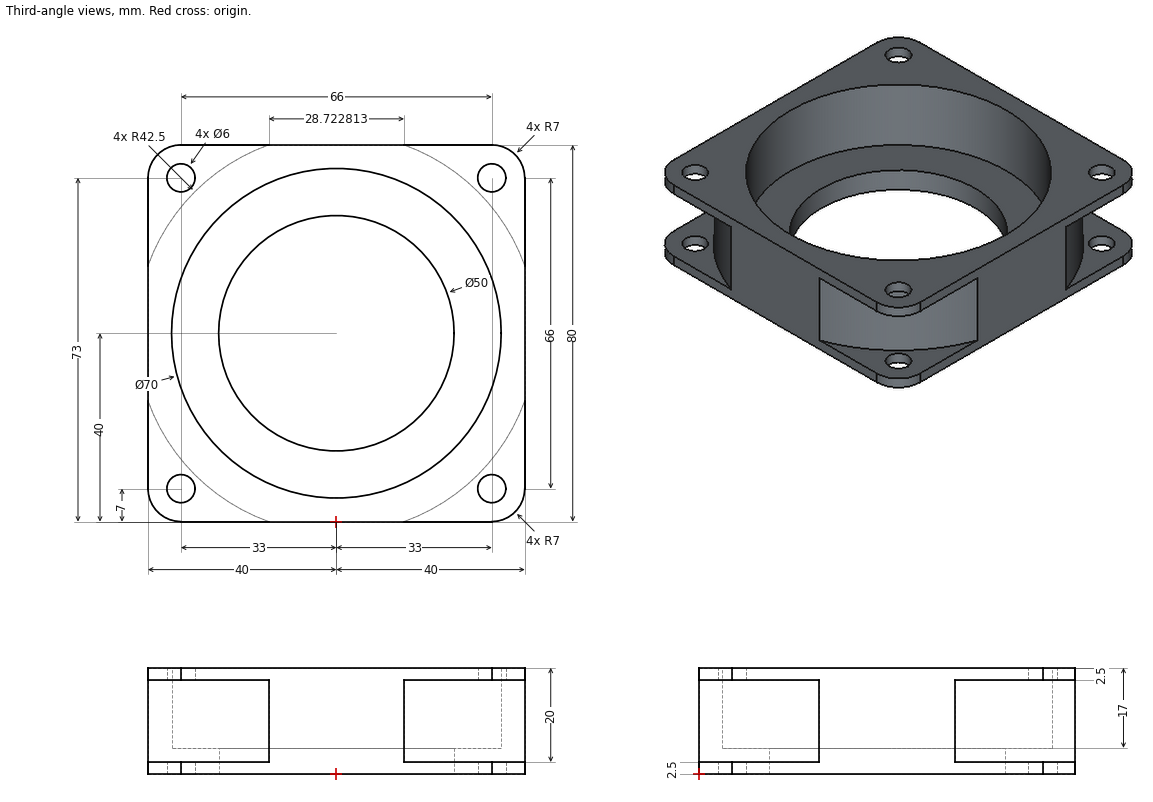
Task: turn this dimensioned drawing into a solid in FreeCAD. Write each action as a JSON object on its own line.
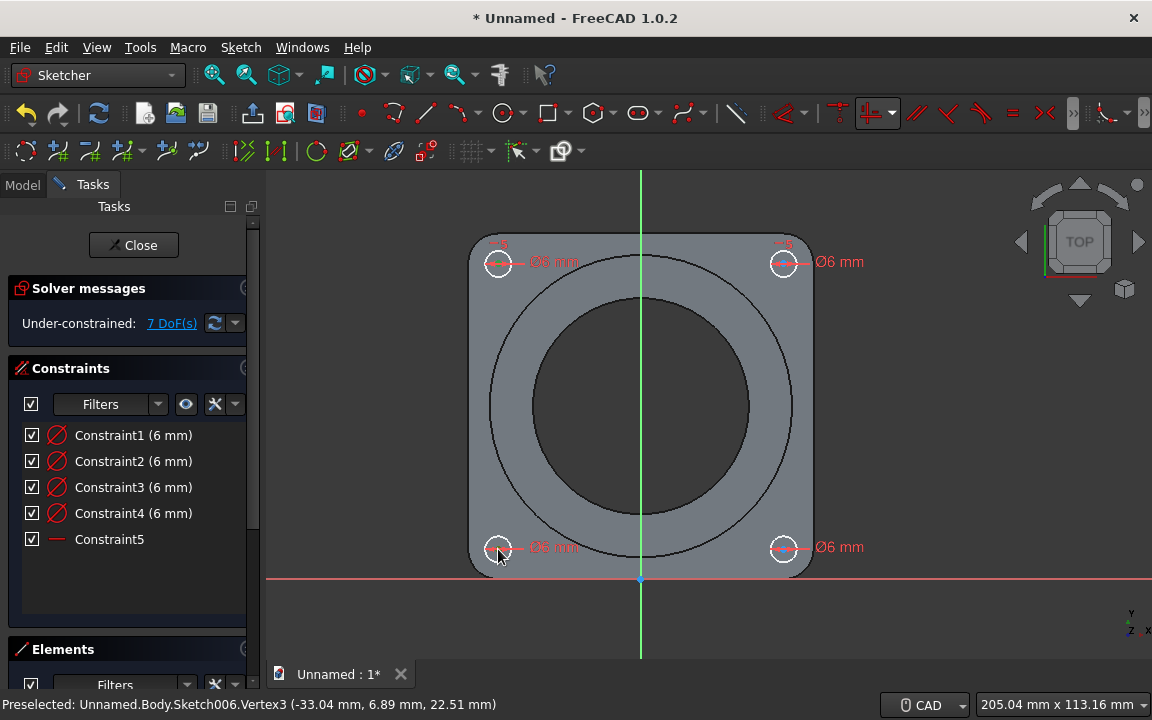
{"action": "left_click", "coordinate": [894, 114]}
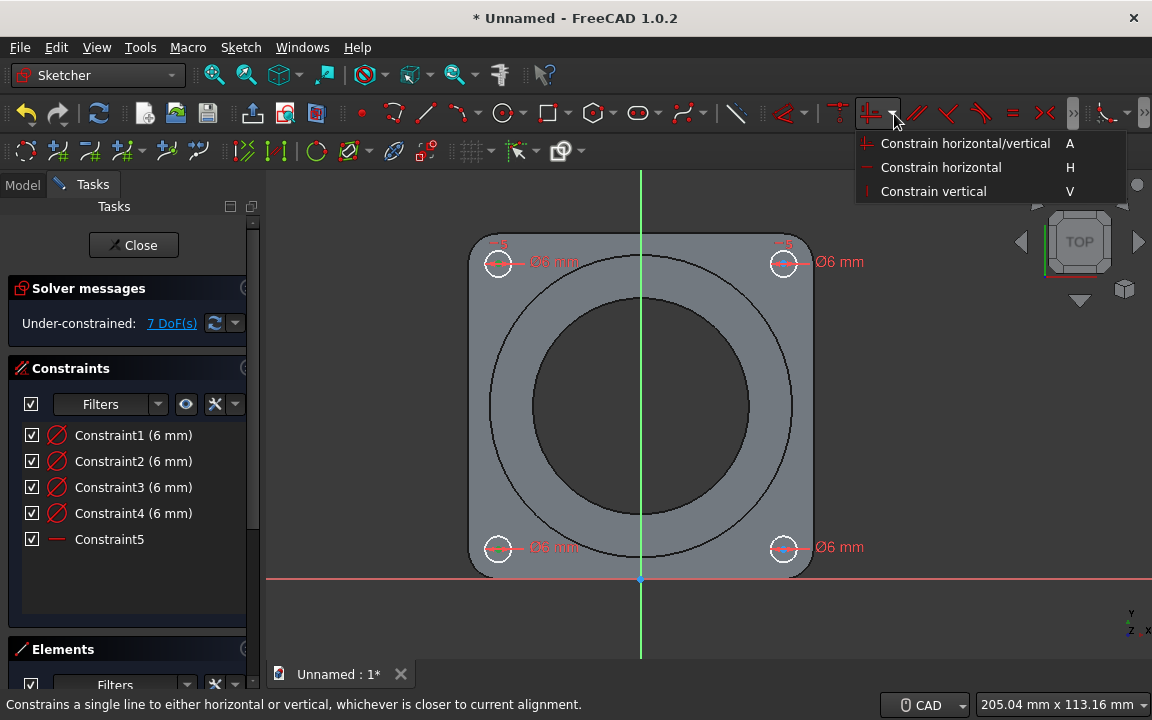
{"action": "left_click", "coordinate": [991, 191]}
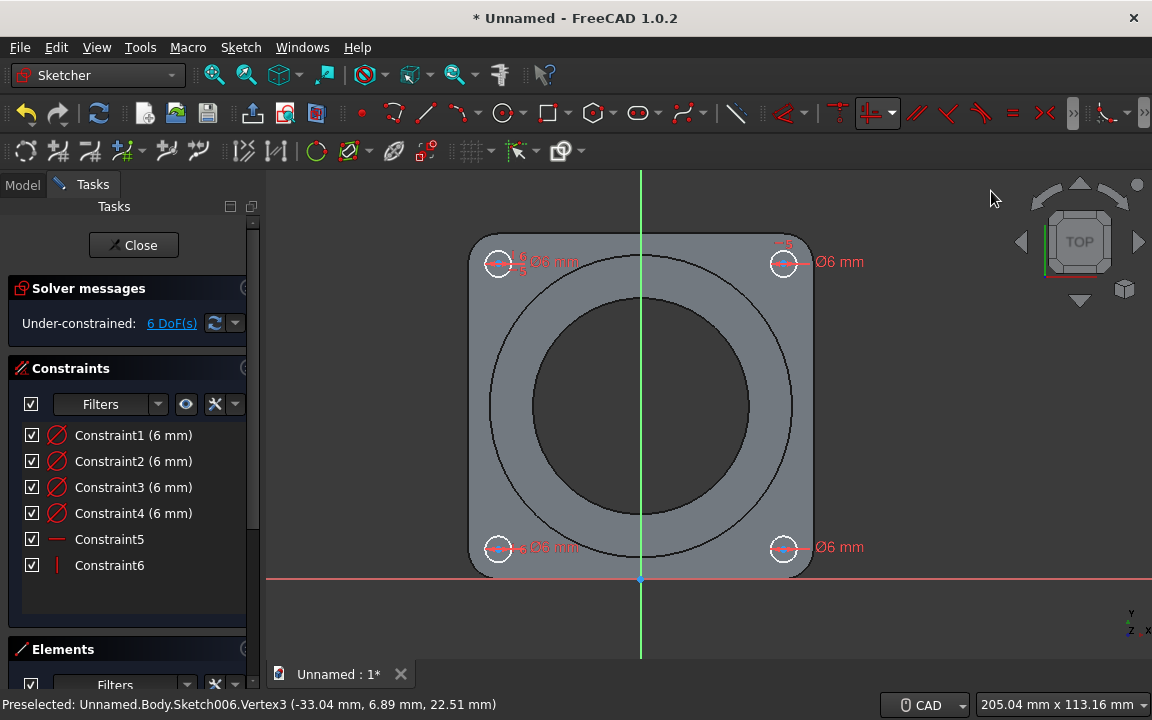
{"action": "left_click", "coordinate": [784, 264]}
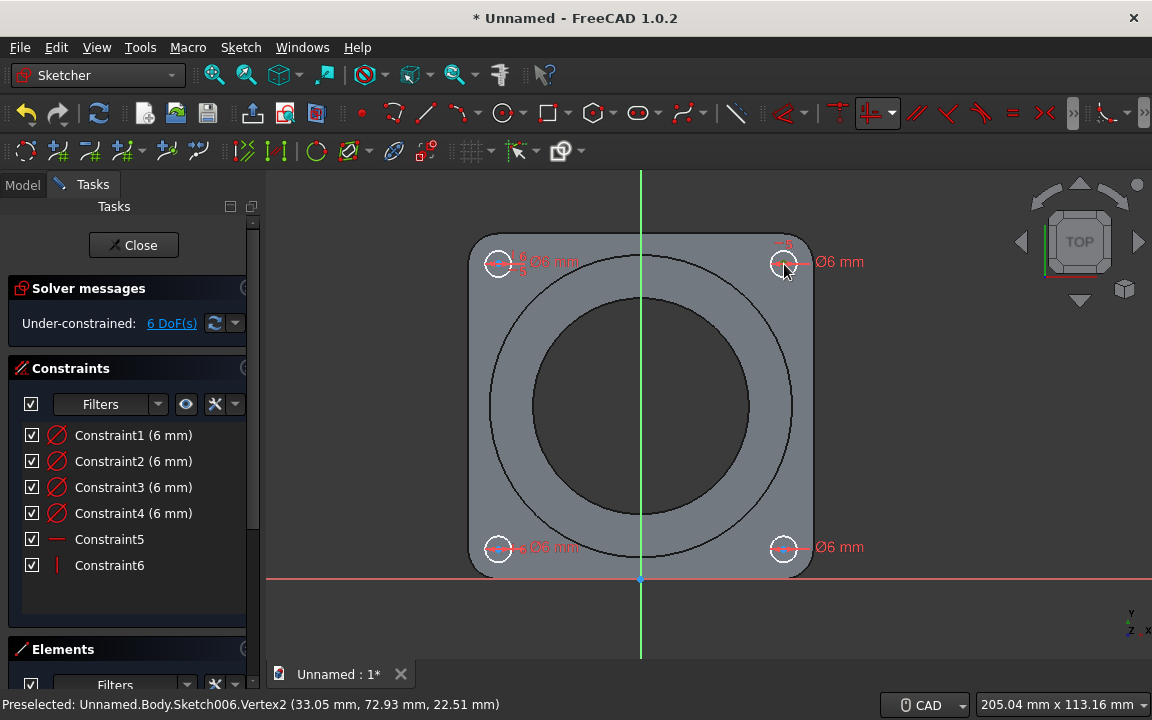
{"action": "left_click", "coordinate": [784, 549]}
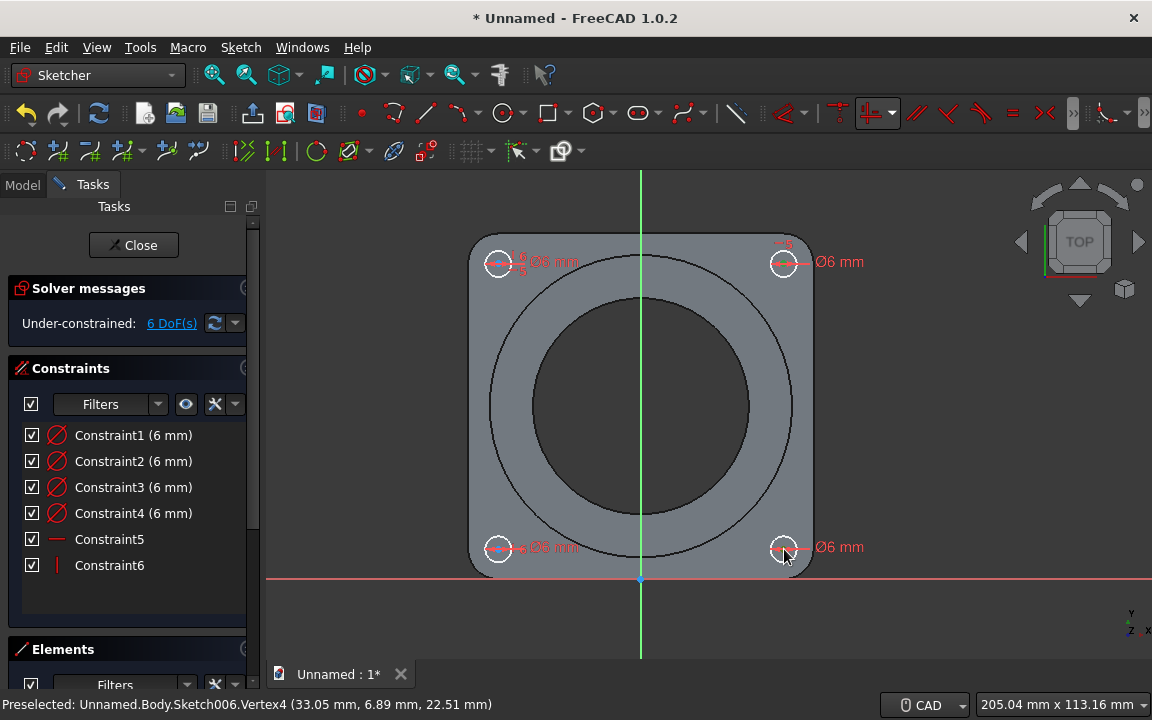
{"action": "key", "text": "v"}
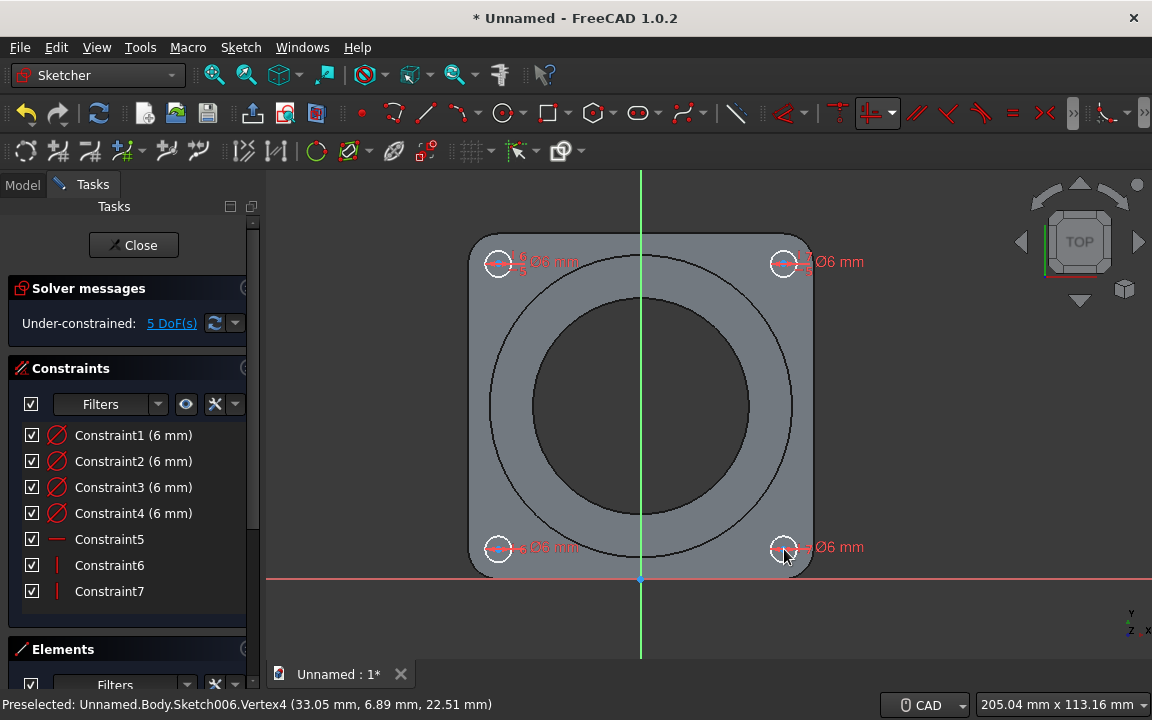
{"action": "left_click", "coordinate": [498, 549]}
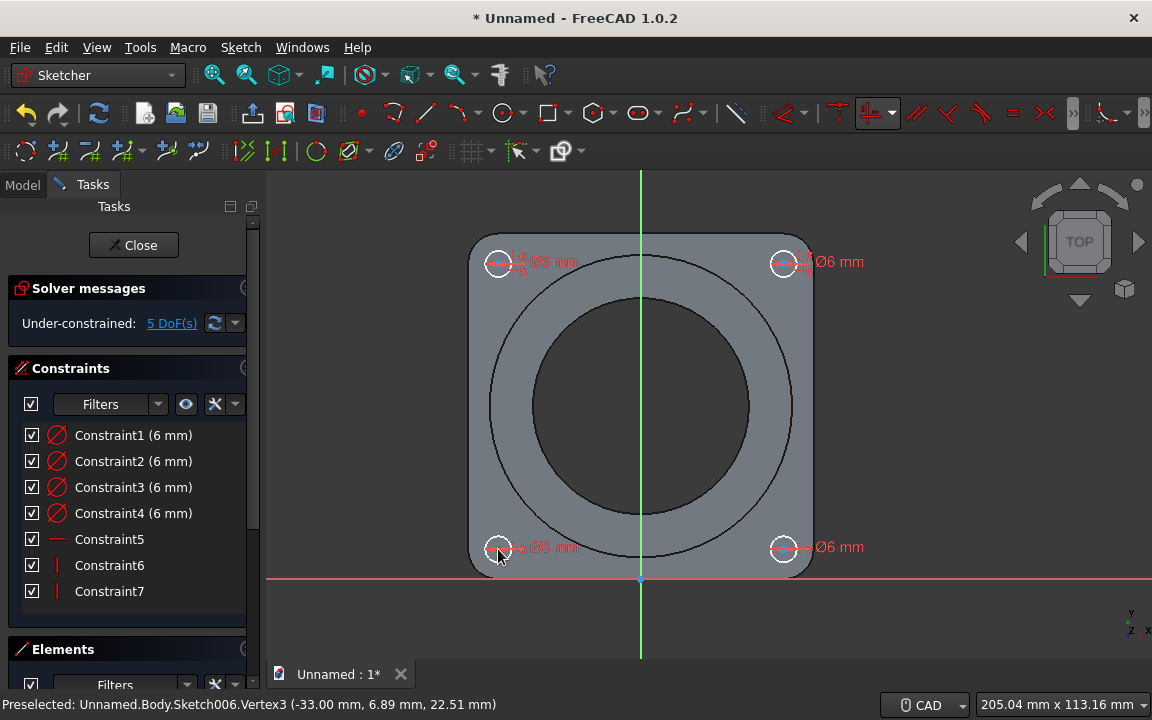
{"action": "left_click", "coordinate": [784, 549]}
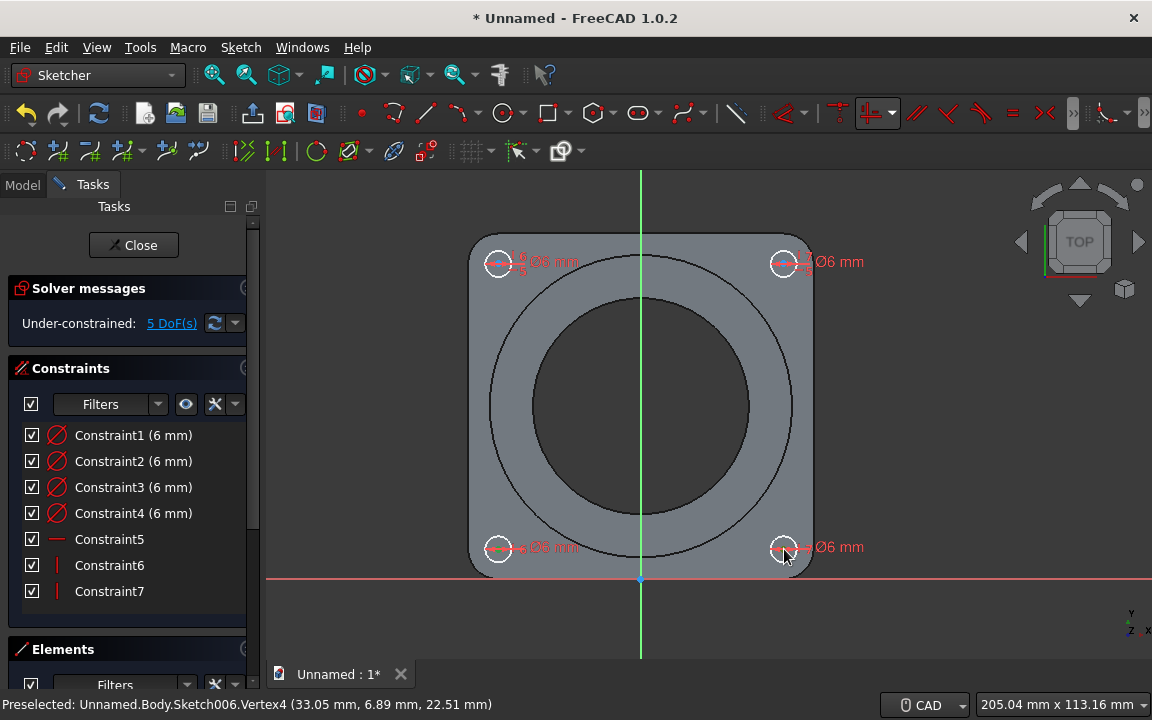
{"action": "key", "text": "h"}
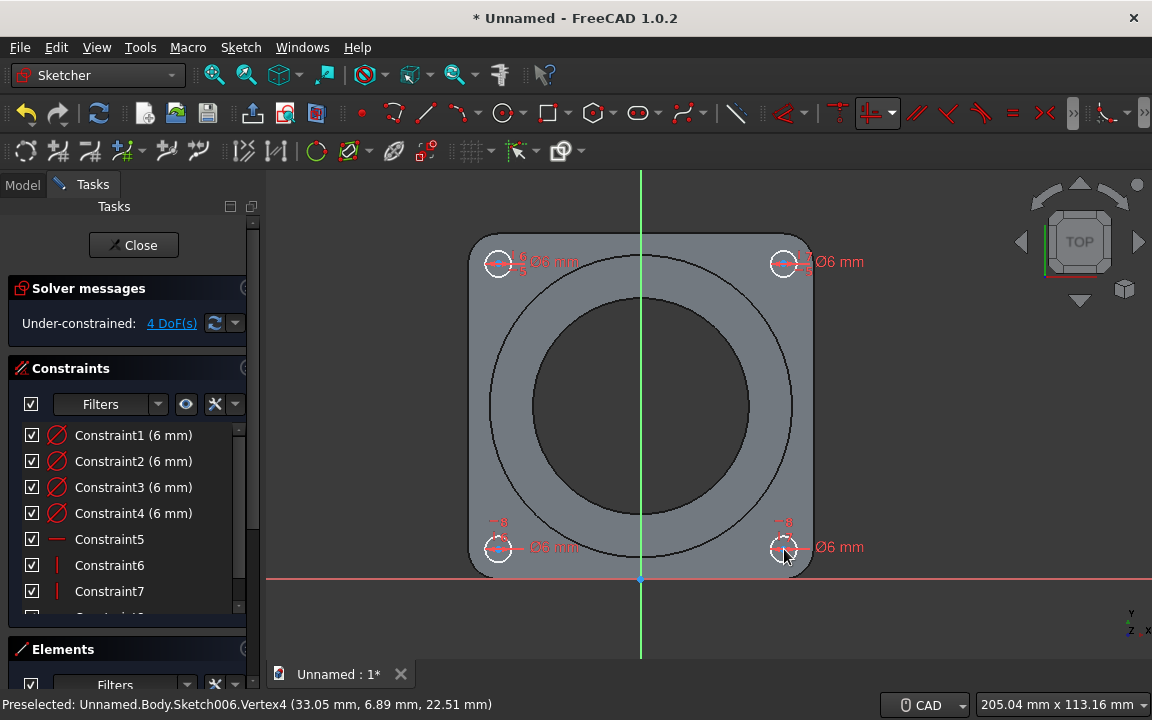
{"action": "key", "text": "d"}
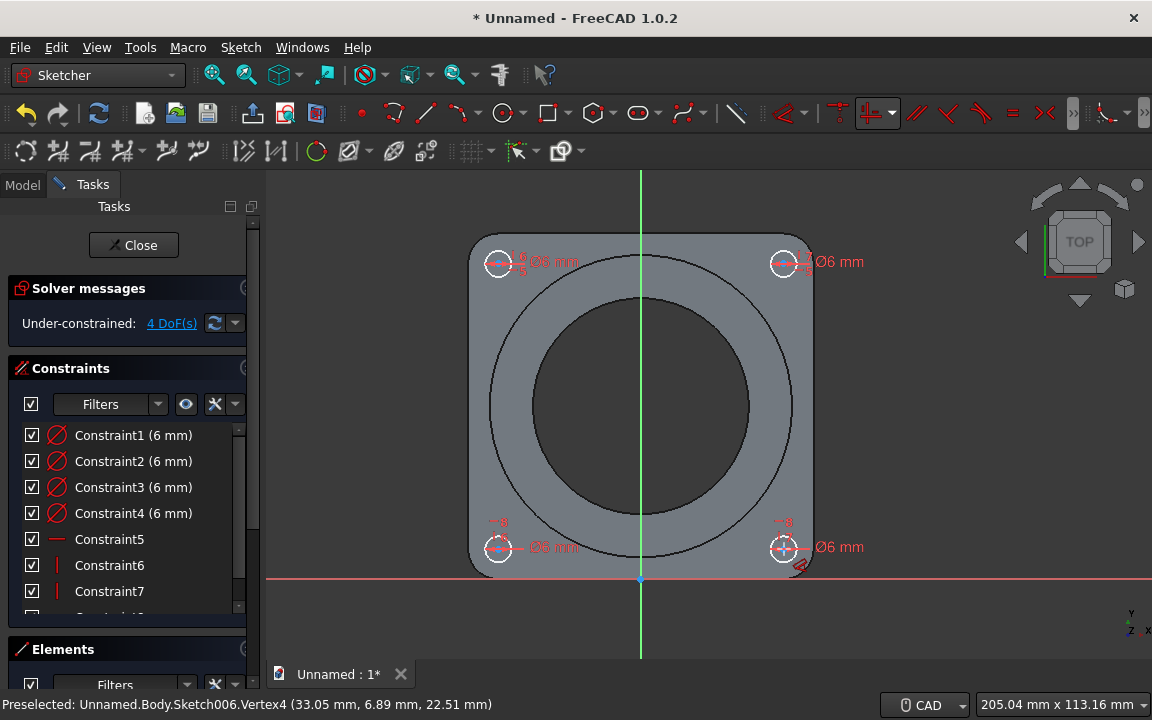
{"action": "scroll", "coordinate": [498, 549], "scroll_direction": "up", "scroll_amount": 2}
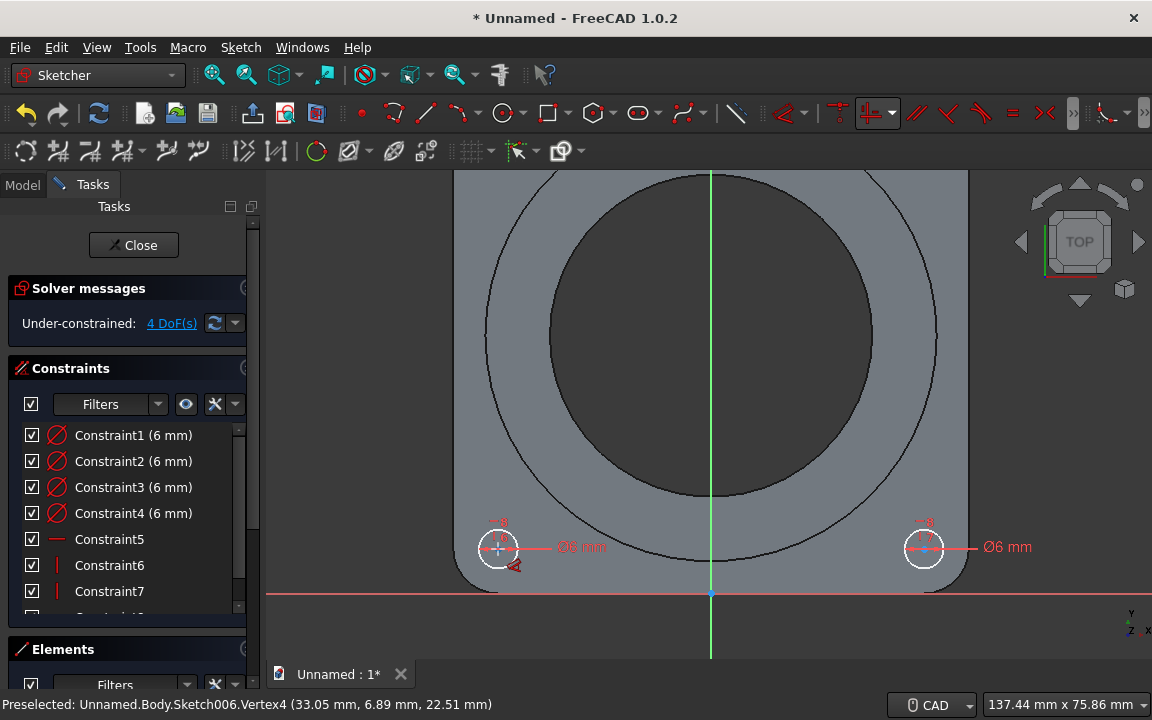
{"action": "left_click", "coordinate": [498, 549]}
{"action": "left_click", "coordinate": [464, 571]}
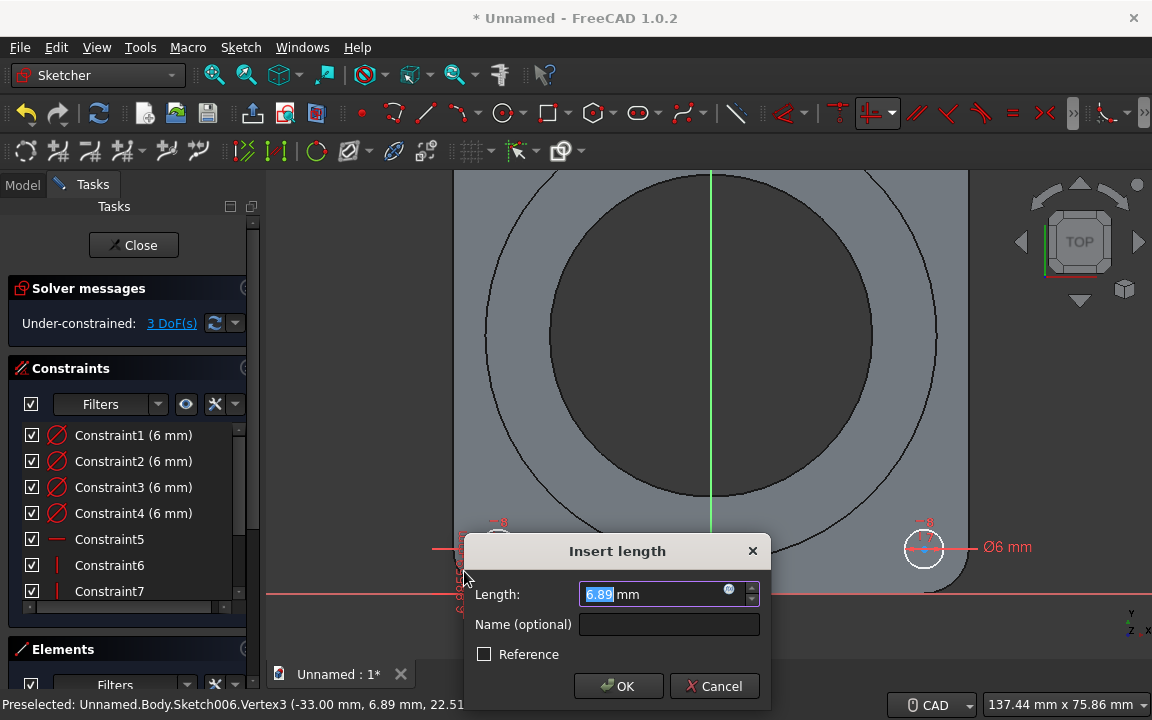
{"action": "type", "text": "7"}
{"action": "key", "text": "Return"}